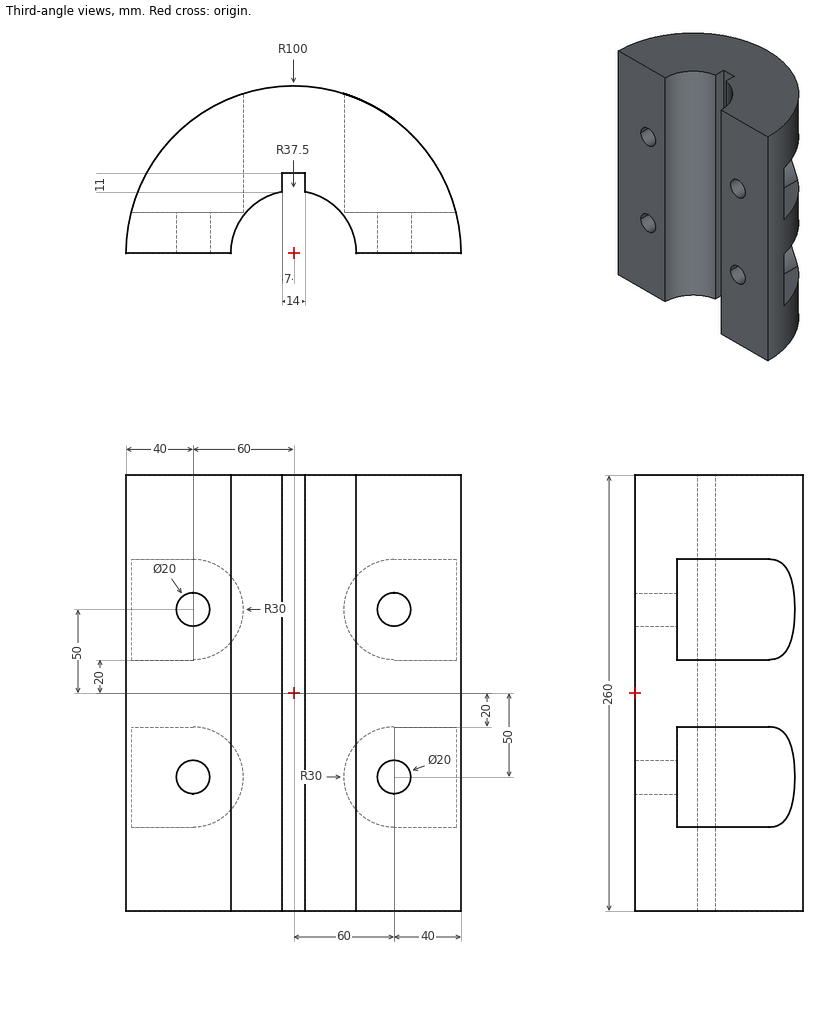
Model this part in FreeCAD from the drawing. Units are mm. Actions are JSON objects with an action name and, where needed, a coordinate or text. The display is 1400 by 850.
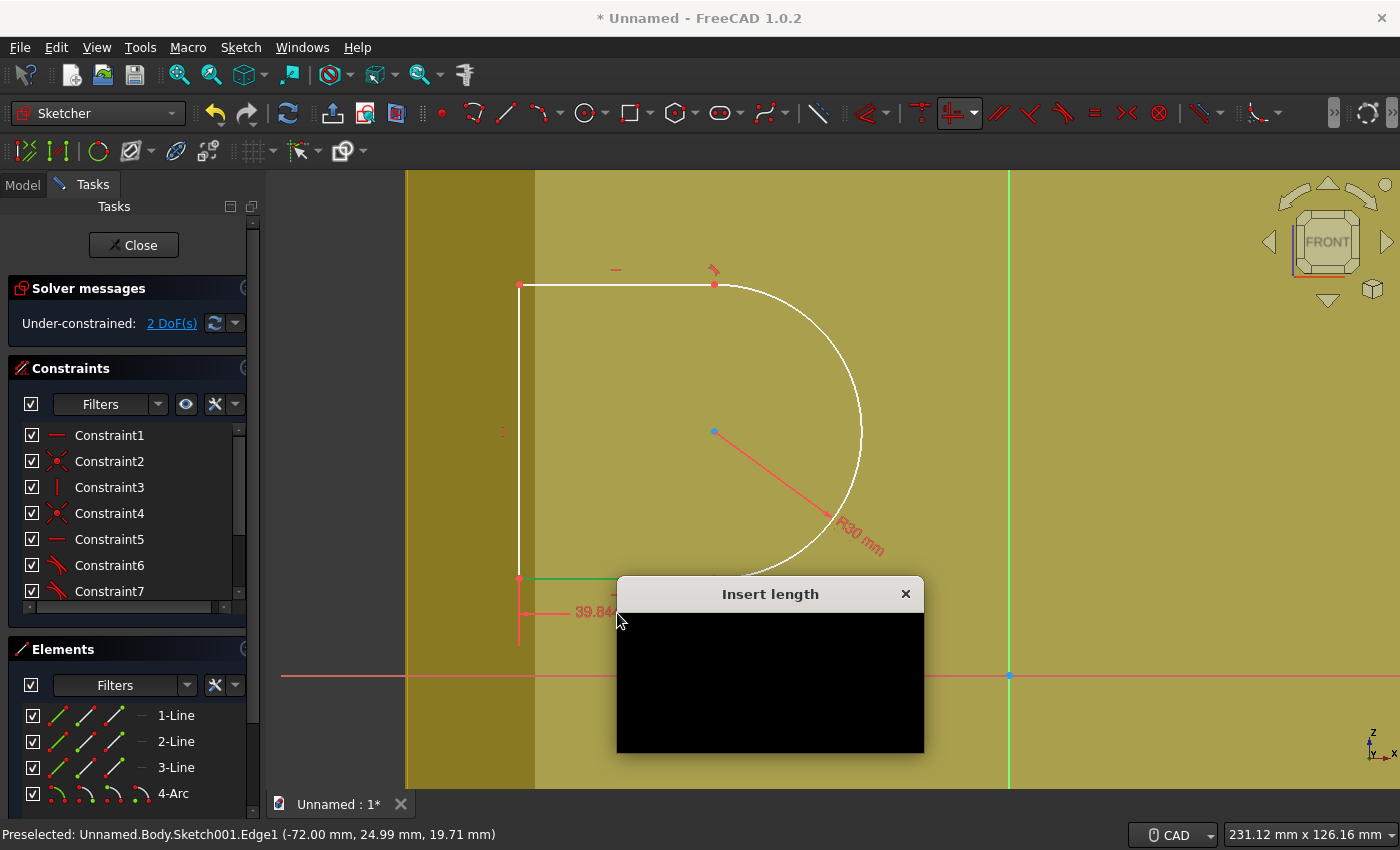
{"action": "type", "text": "40"}
{"action": "key", "text": "Return"}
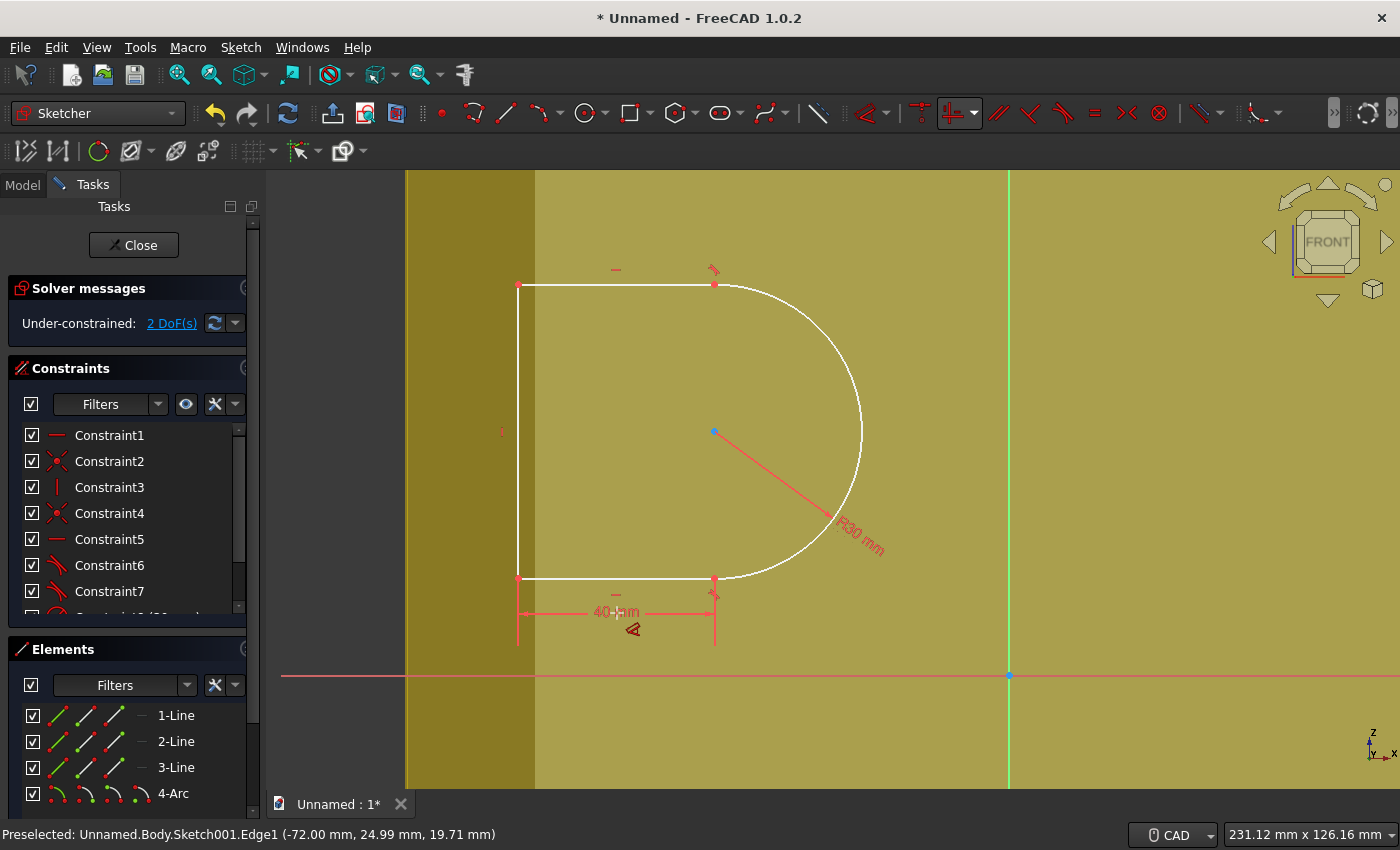
{"action": "left_click", "coordinate": [715, 579]}
{"action": "left_click", "coordinate": [862, 710]}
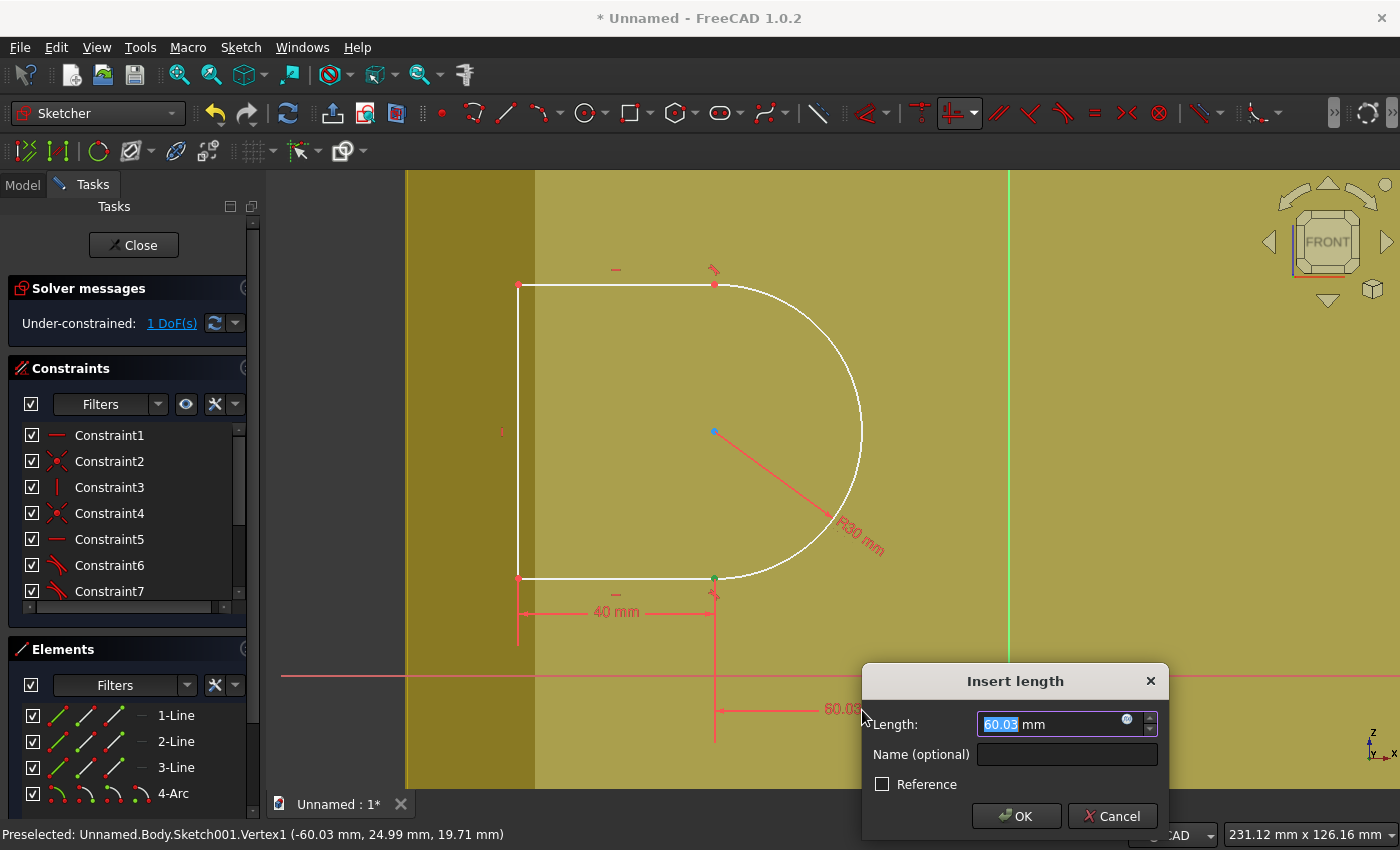
{"action": "type", "text": "60"}
{"action": "key", "text": "Return"}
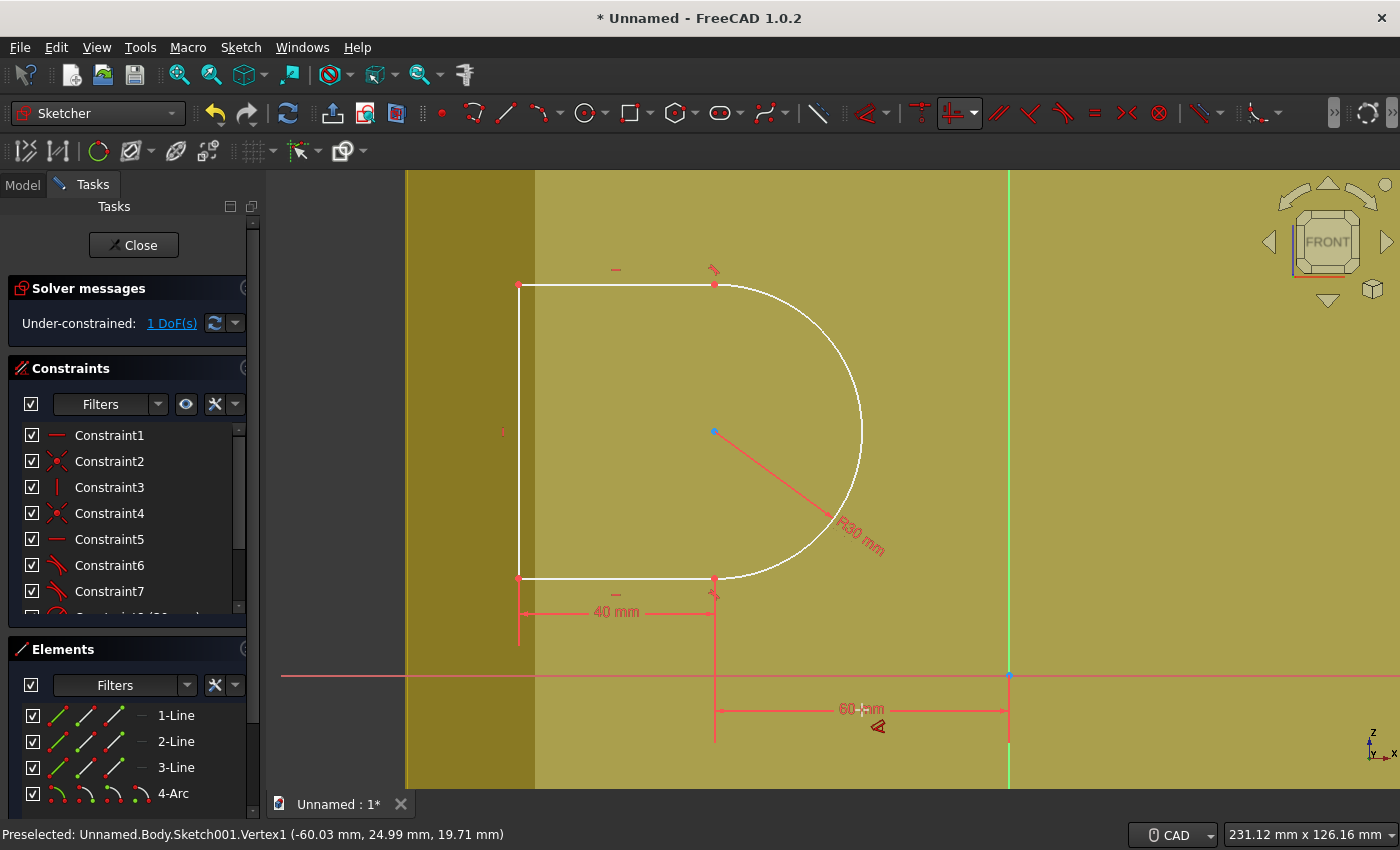
{"action": "left_click", "coordinate": [715, 579]}
{"action": "left_click", "coordinate": [1043, 627]}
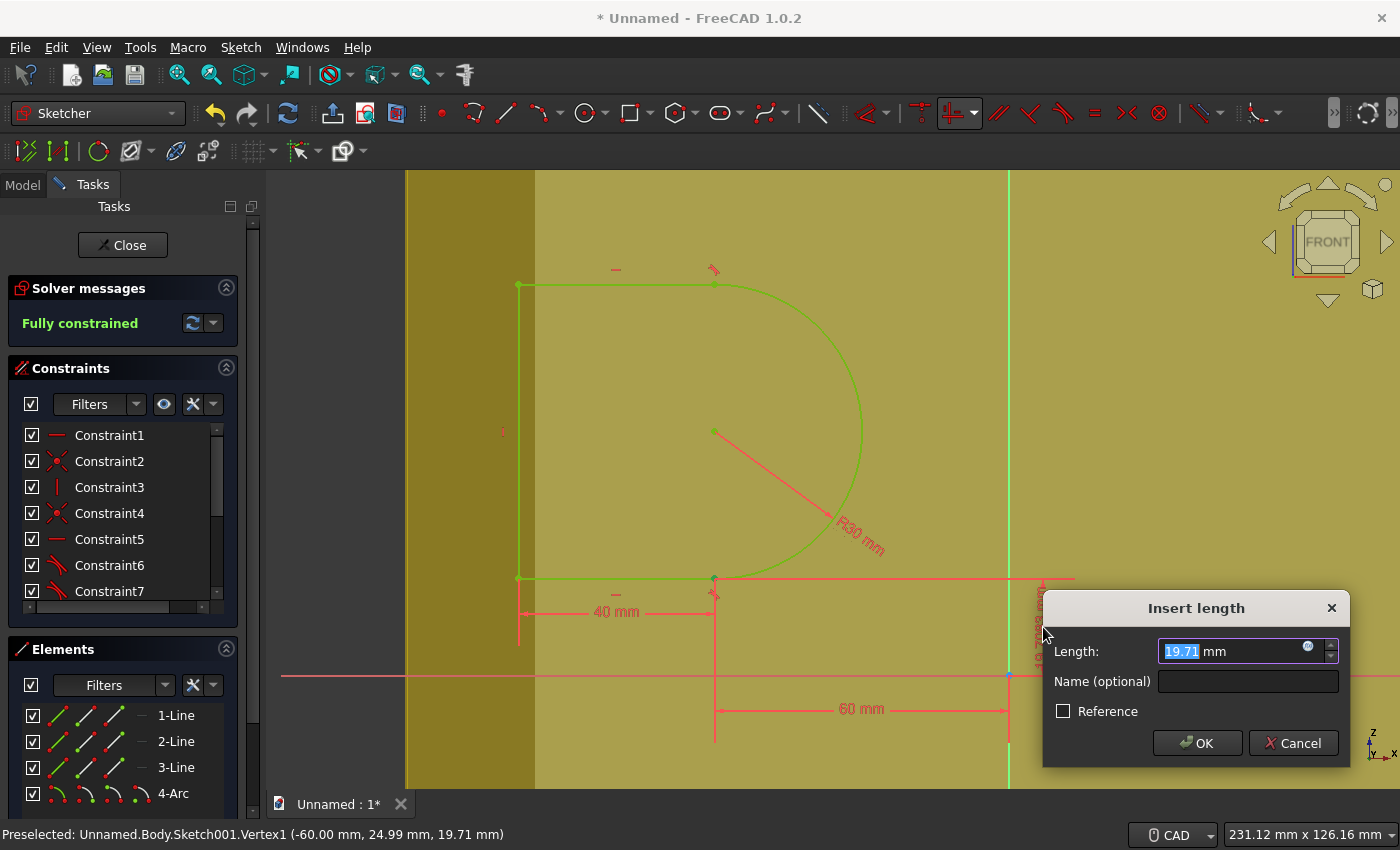
{"action": "type", "text": "20"}
{"action": "key", "text": "Return"}
{"action": "key", "text": "Escape"}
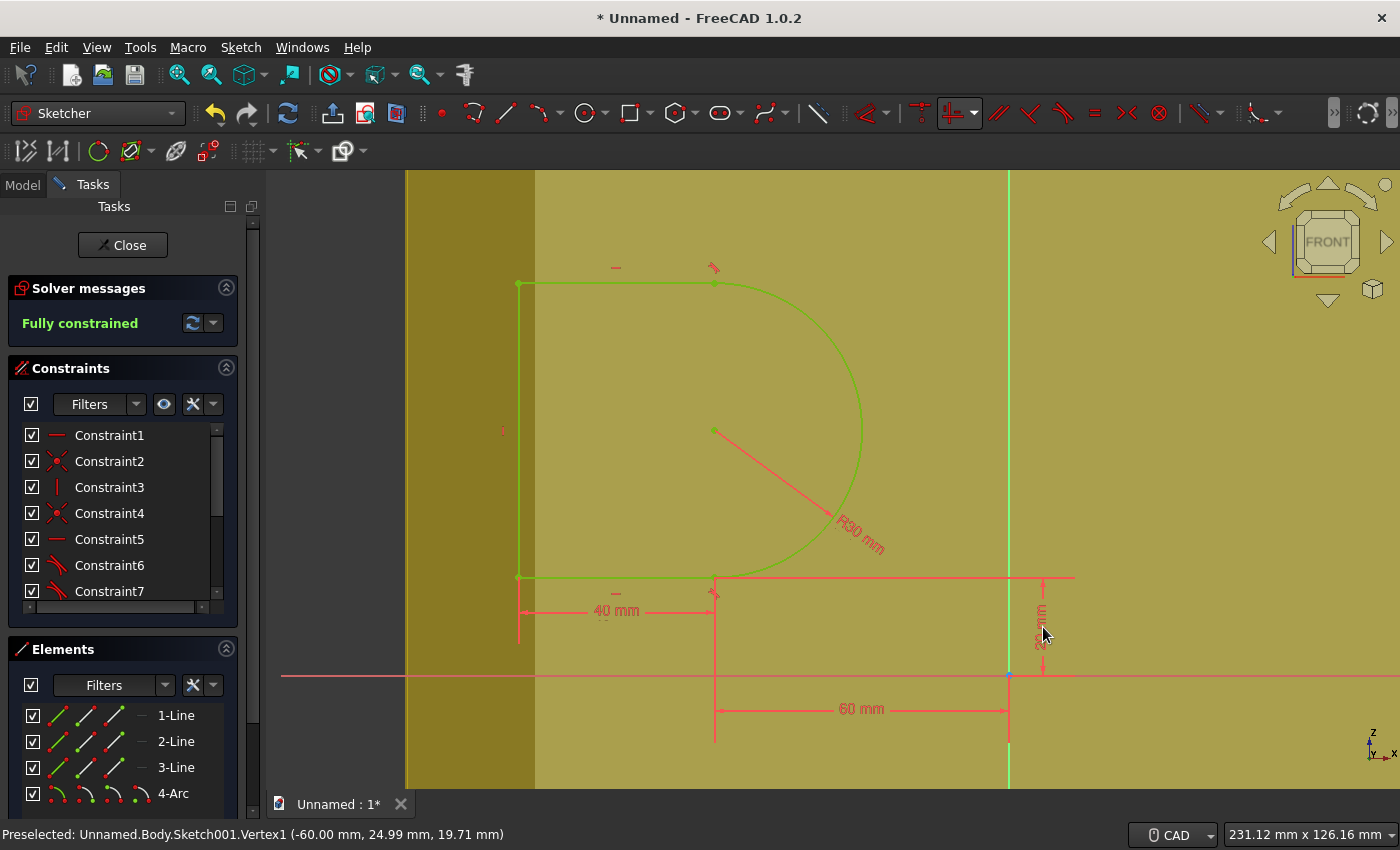
{"action": "left_click", "coordinate": [123, 245]}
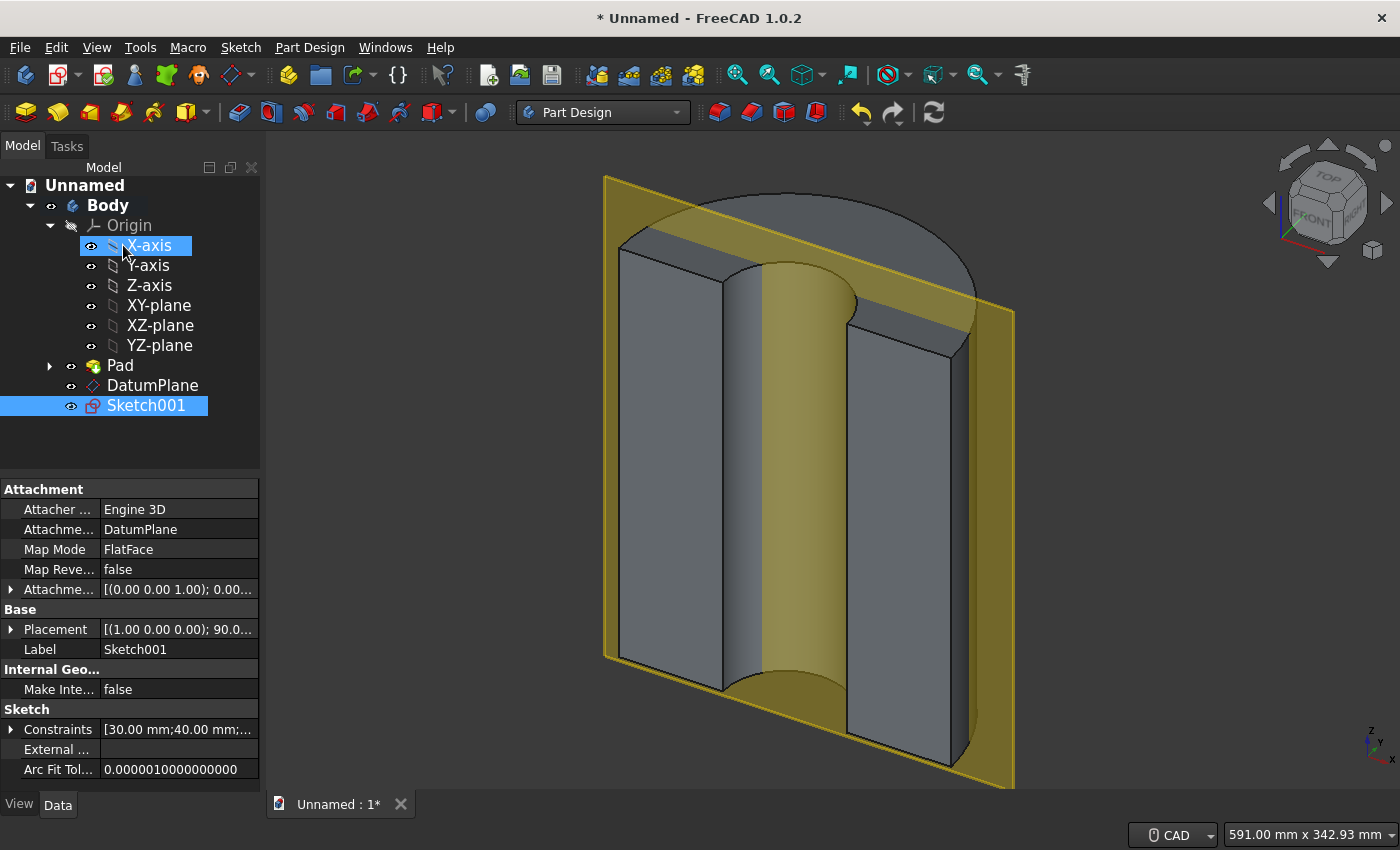
{"action": "left_click", "coordinate": [240, 112]}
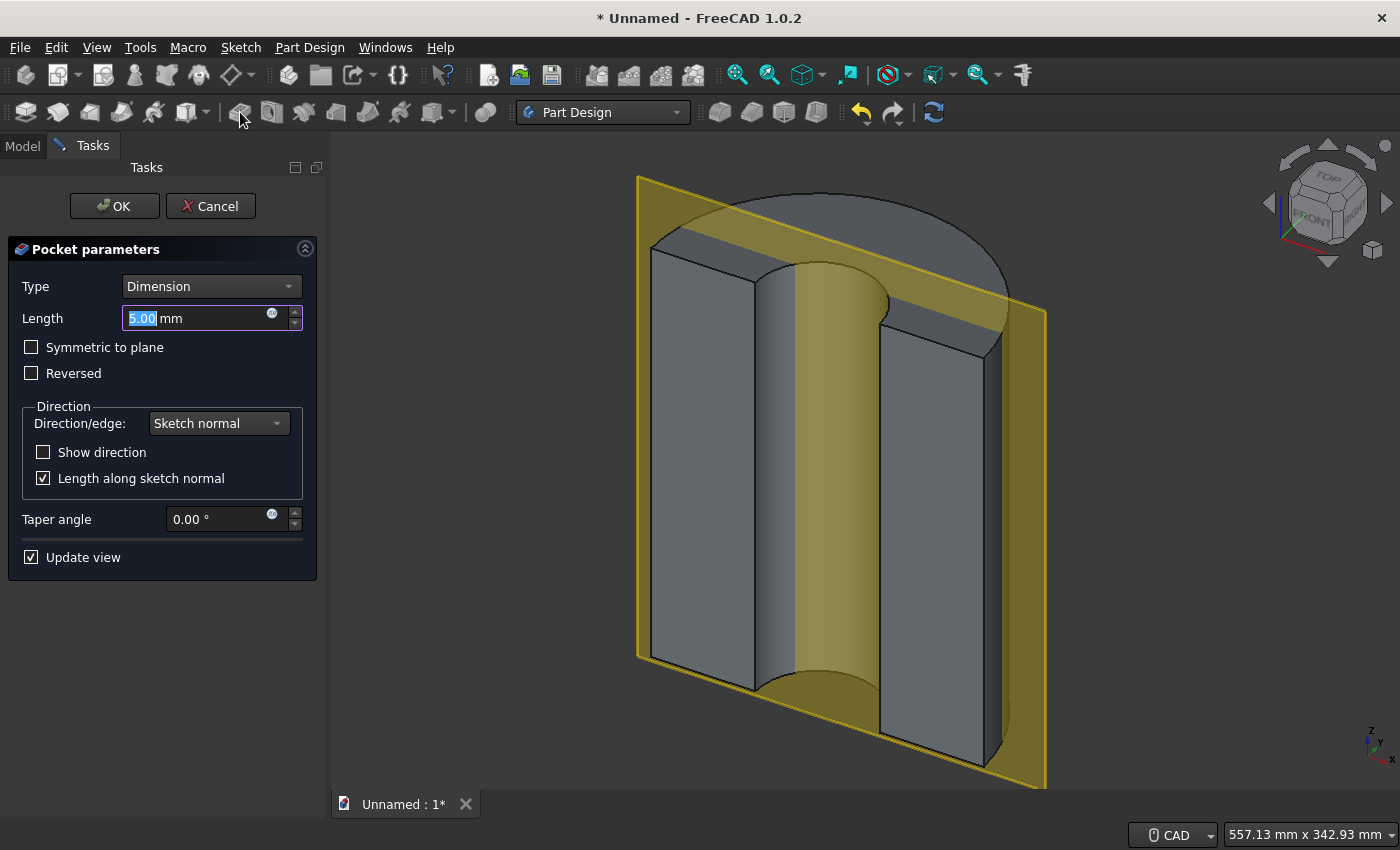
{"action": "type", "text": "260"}
{"action": "key", "text": "Tab"}